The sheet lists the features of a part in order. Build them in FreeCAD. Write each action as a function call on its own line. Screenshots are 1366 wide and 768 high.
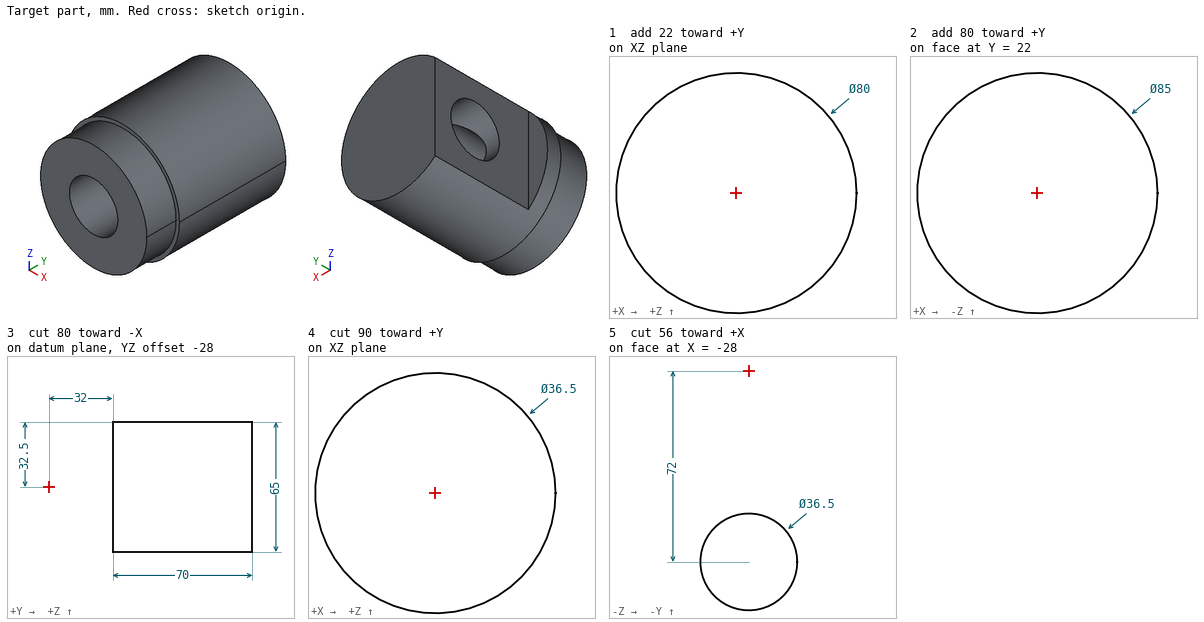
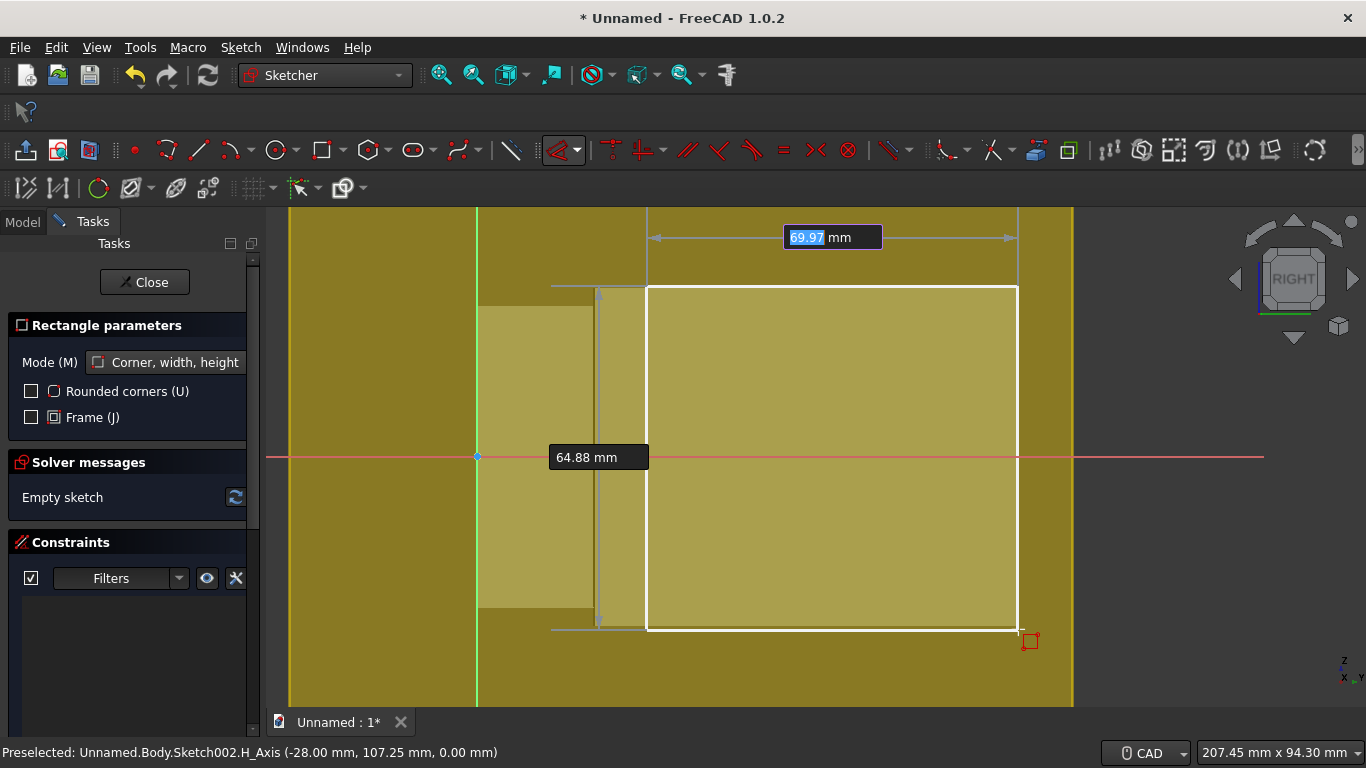
text(70)
key(Tab)
text(65)
key(Return)
key(Escape)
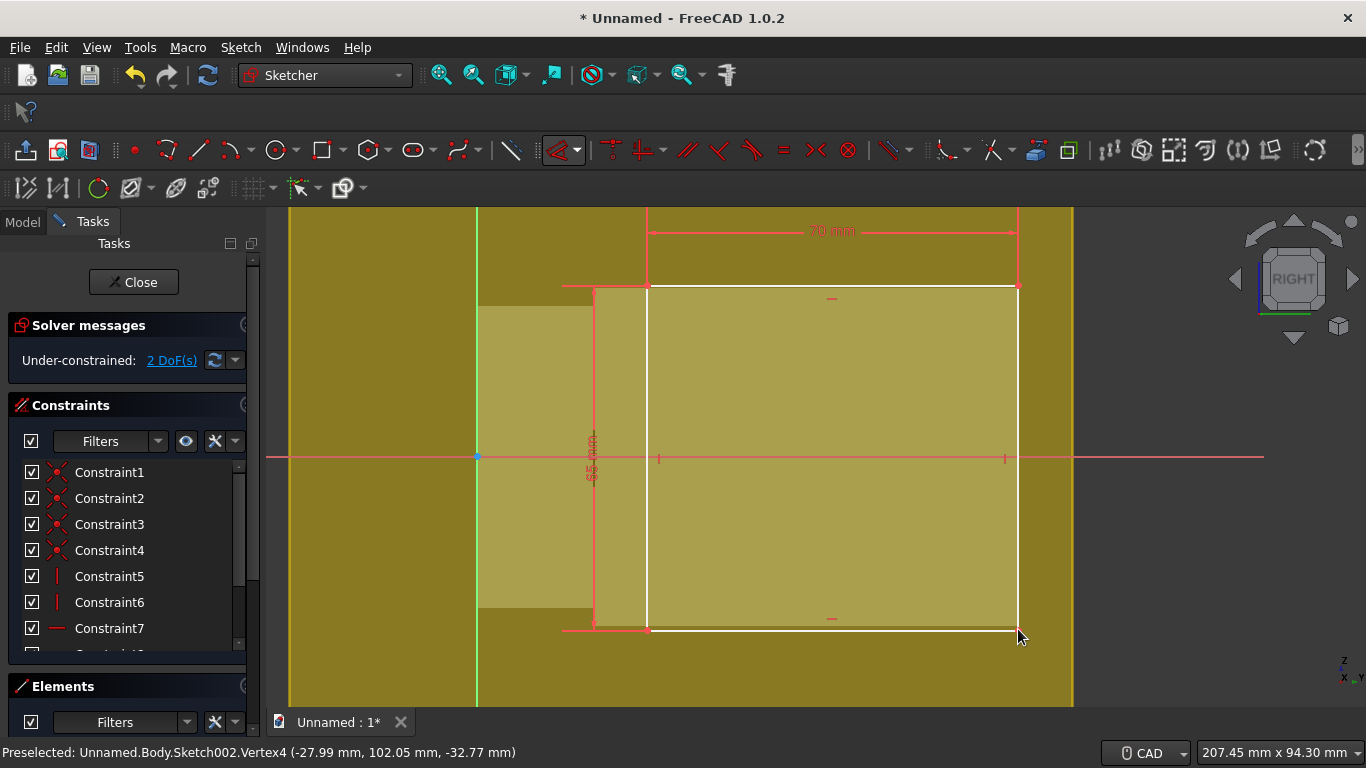
click(647, 286)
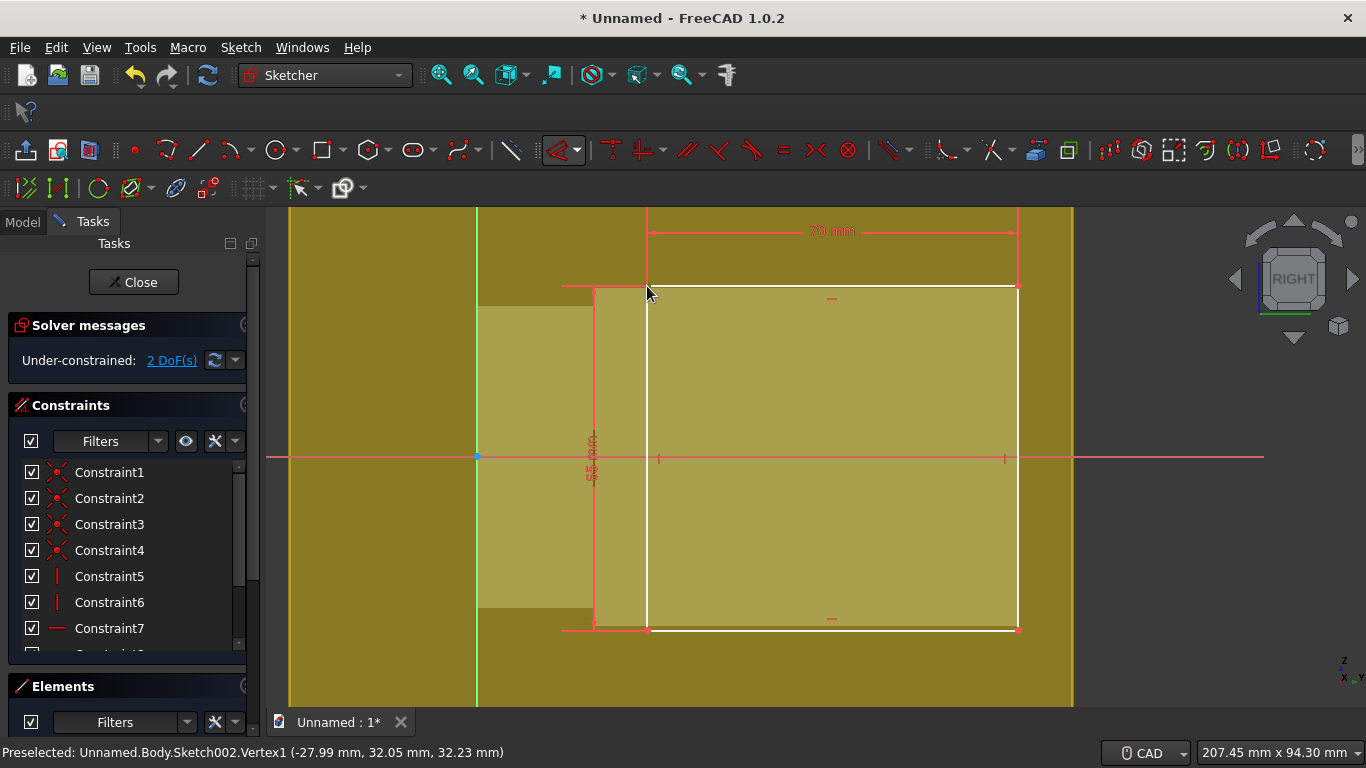
click(580, 150)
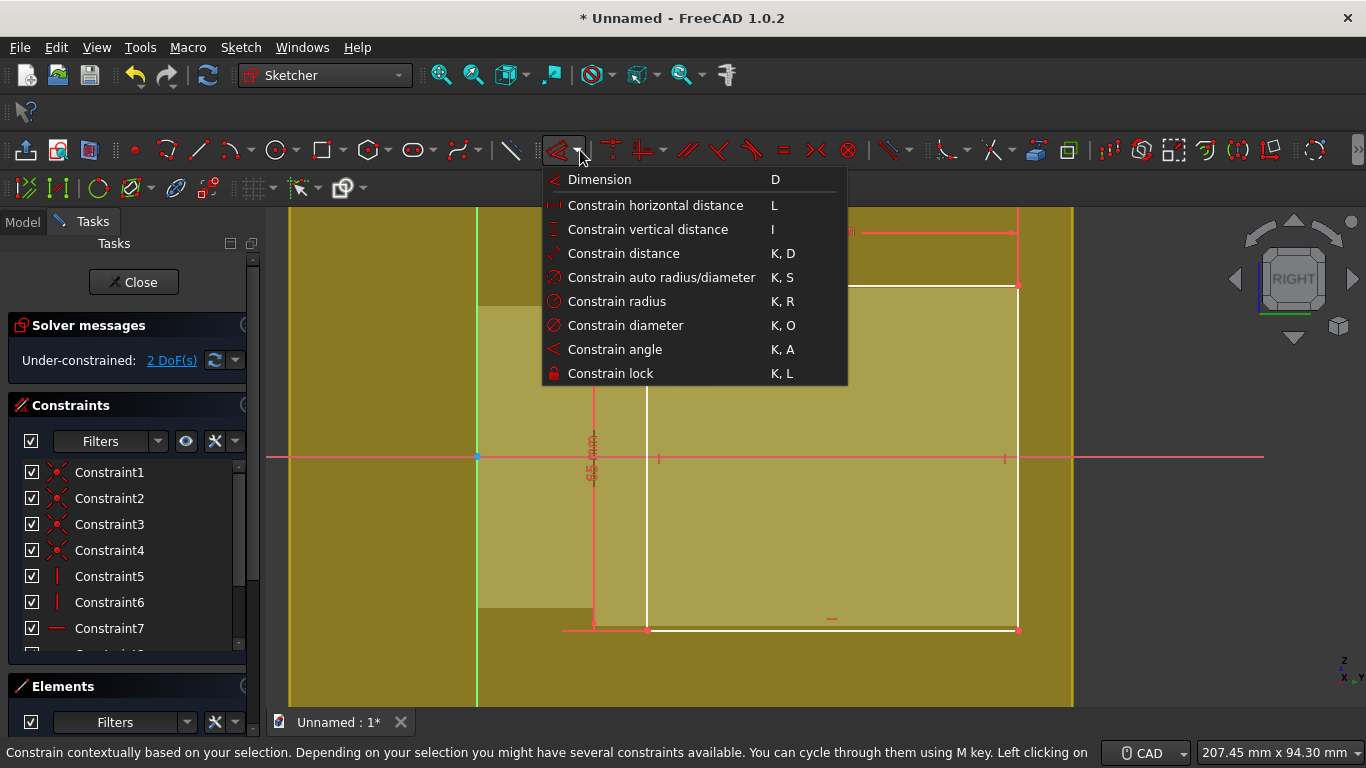
click(695, 205)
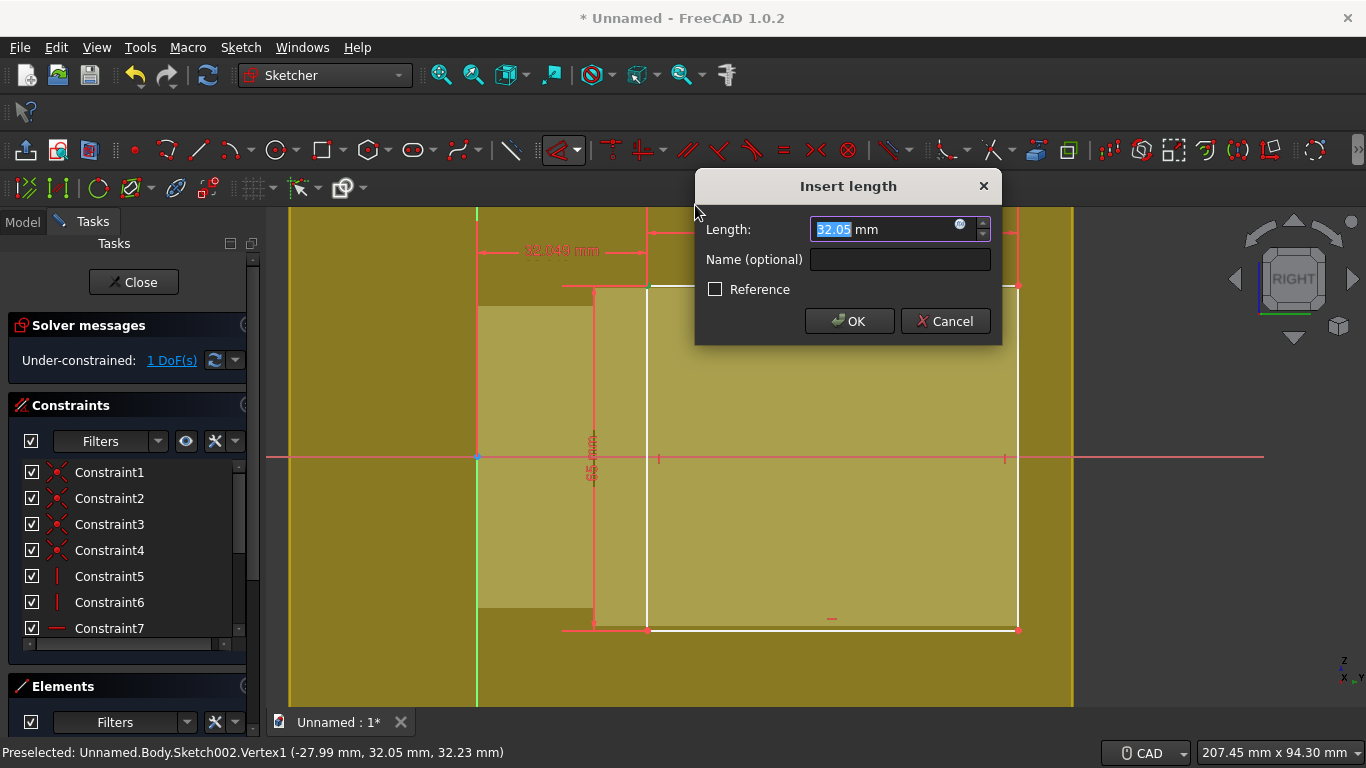
text(32)
key(Return)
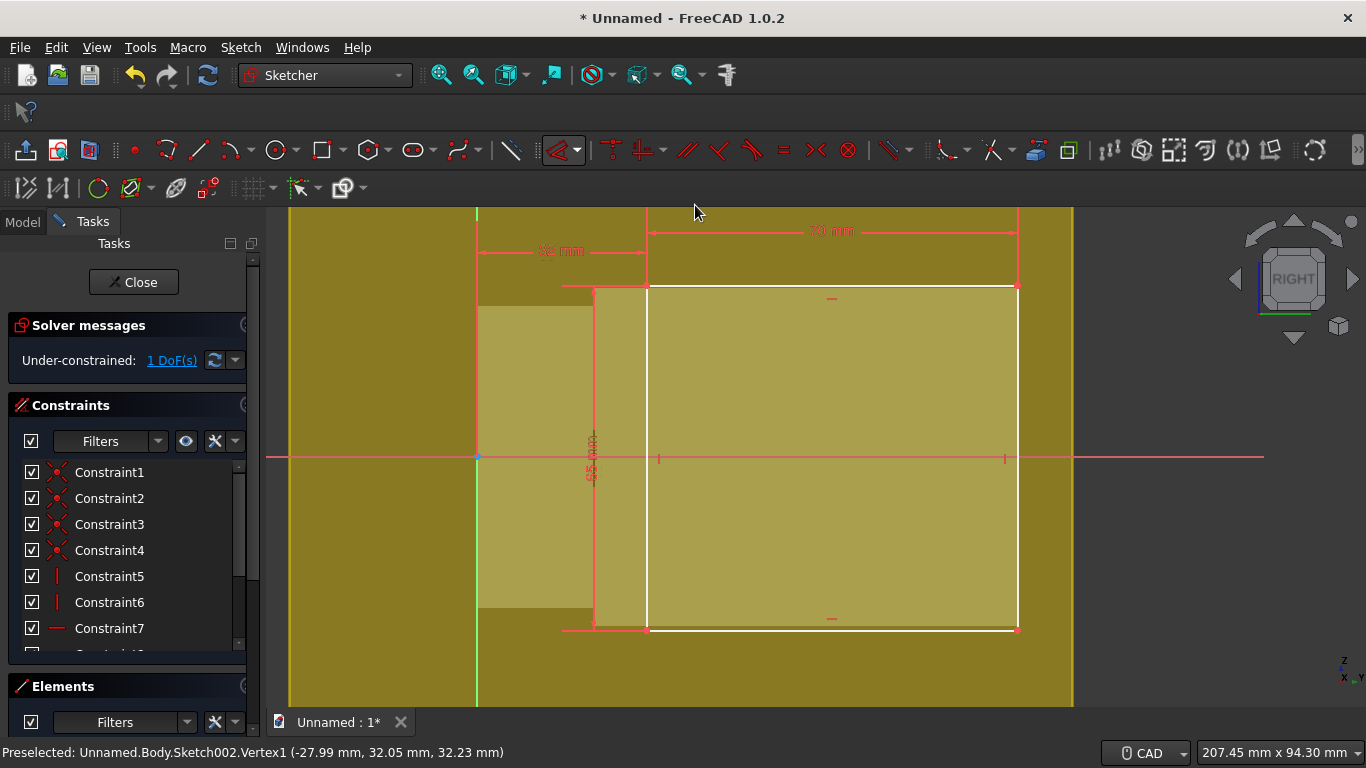
click(647, 286)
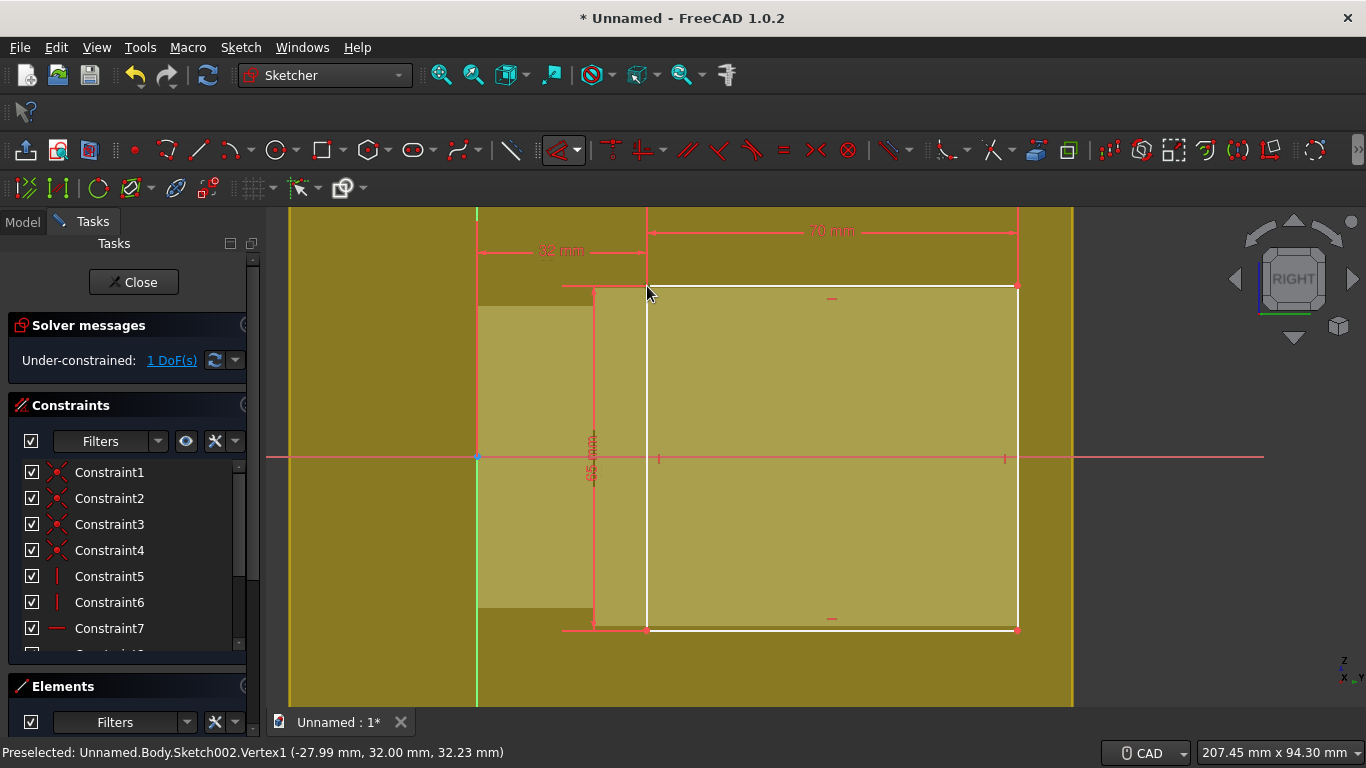
key(i)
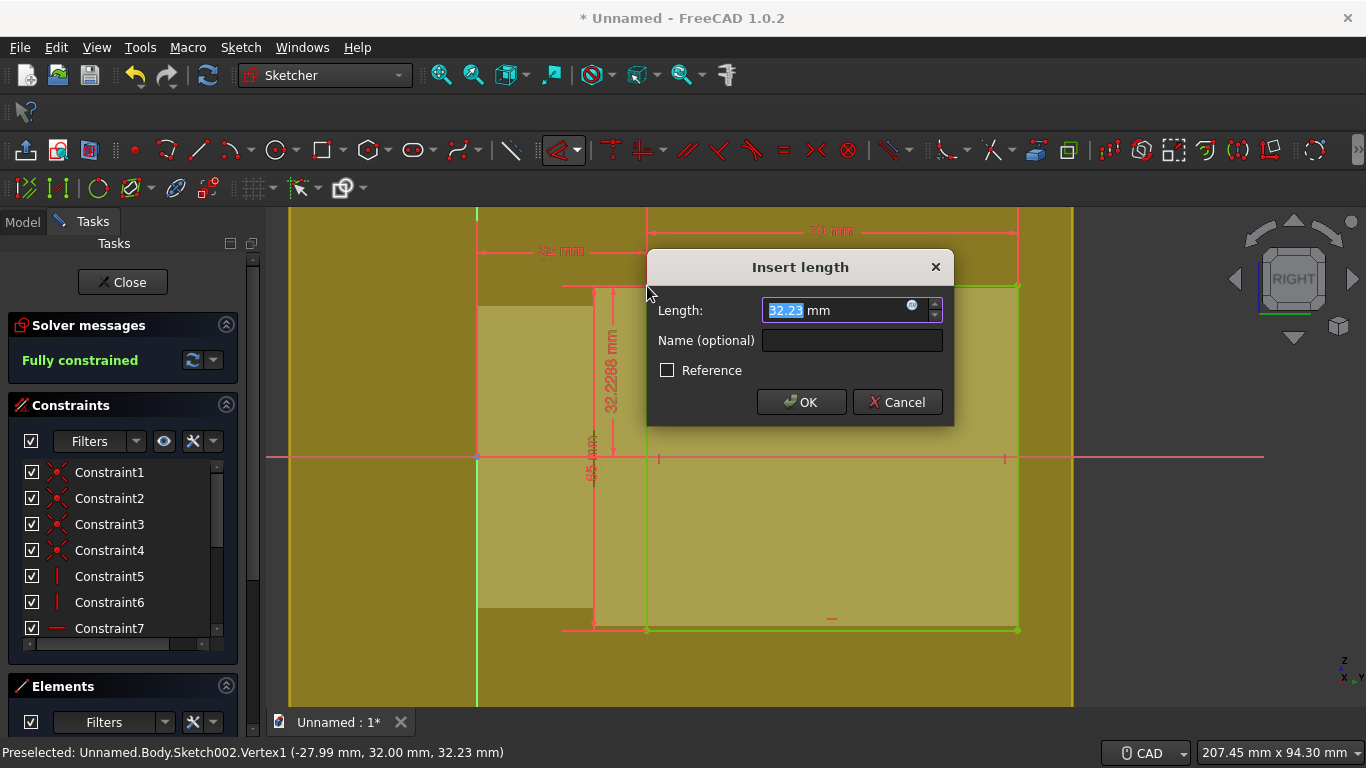
text(32.5)
key(Return)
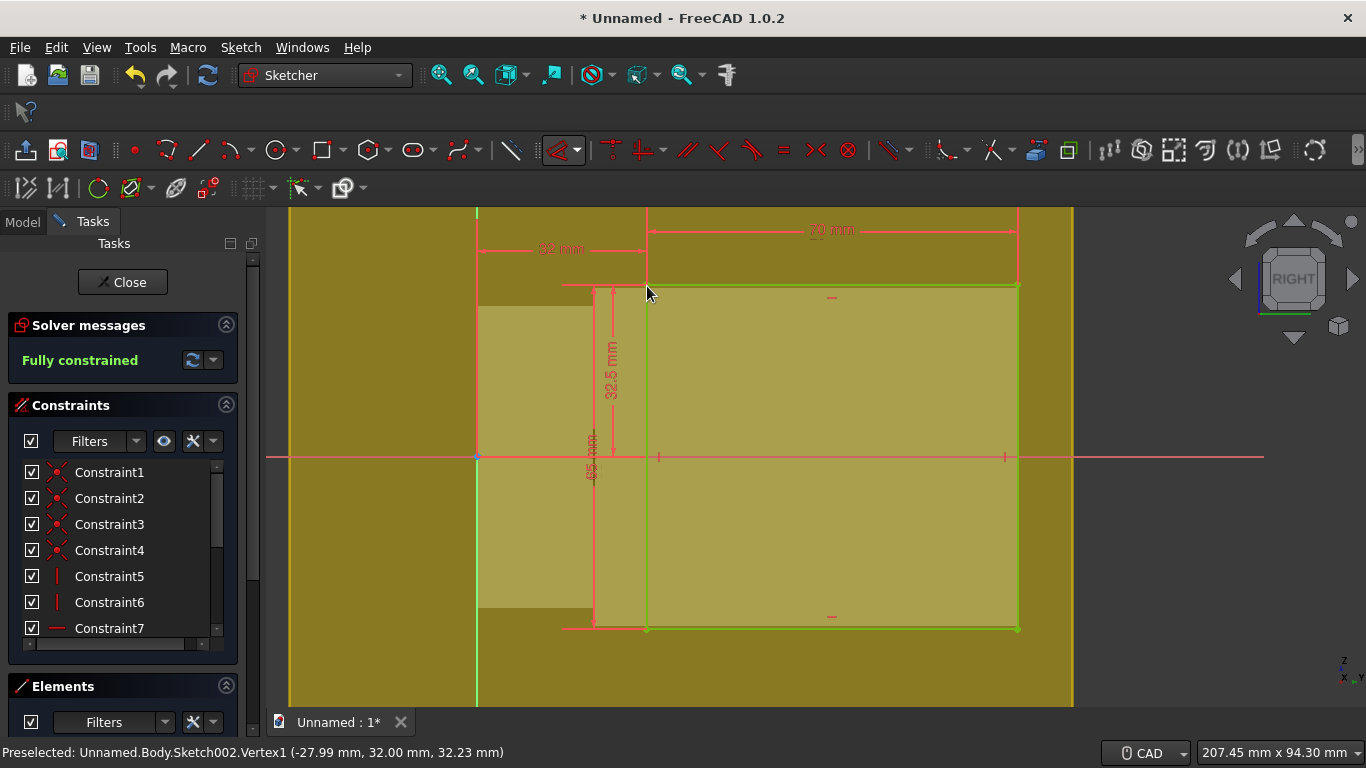
click(123, 282)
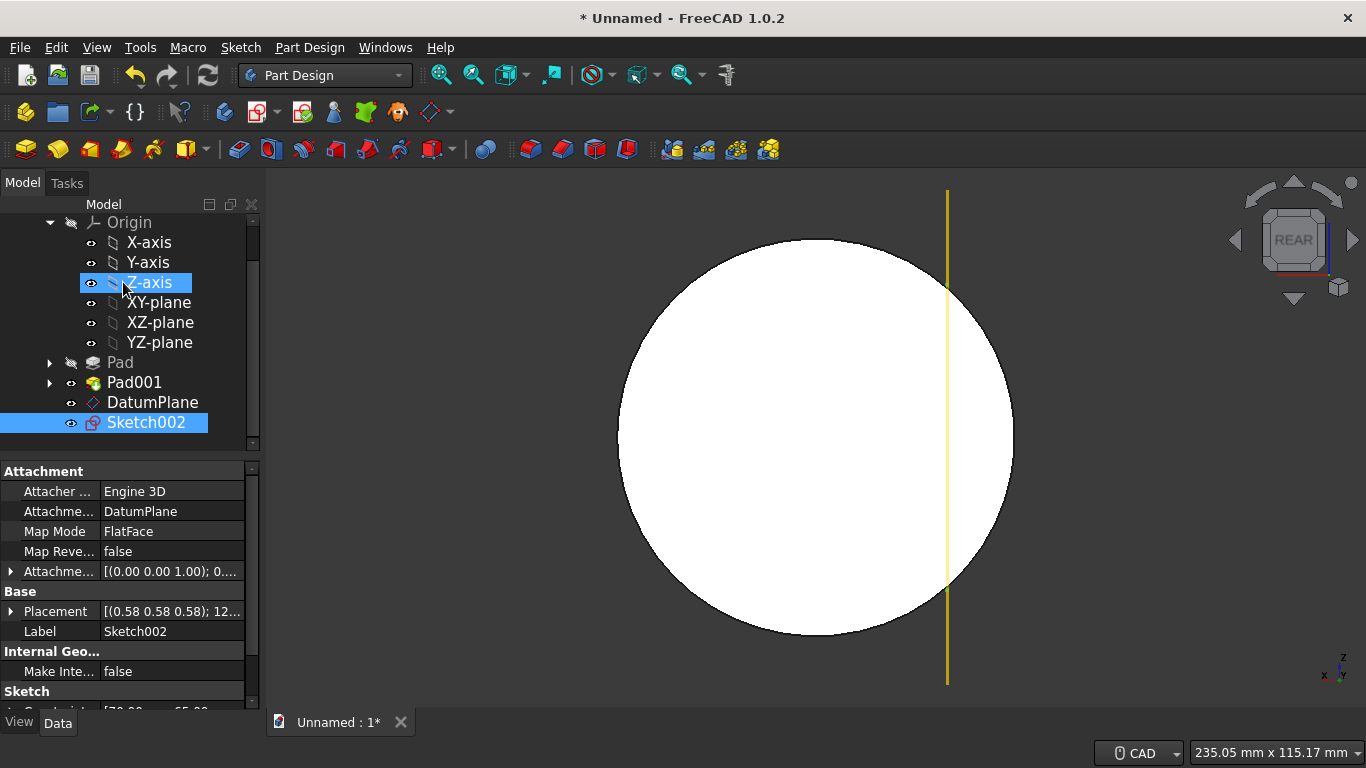
click(240, 150)